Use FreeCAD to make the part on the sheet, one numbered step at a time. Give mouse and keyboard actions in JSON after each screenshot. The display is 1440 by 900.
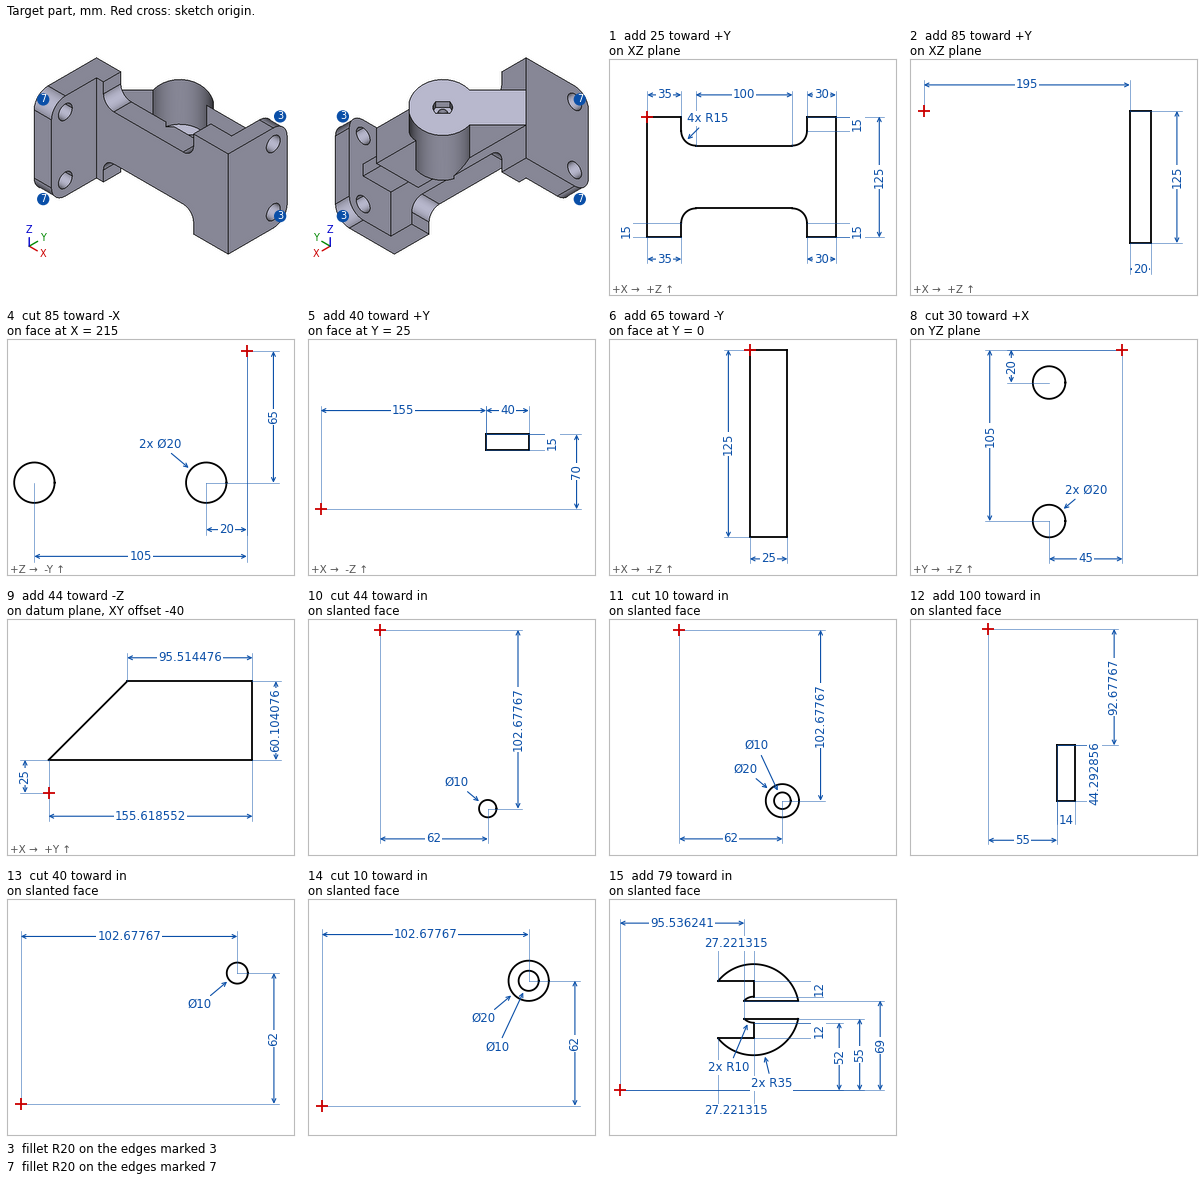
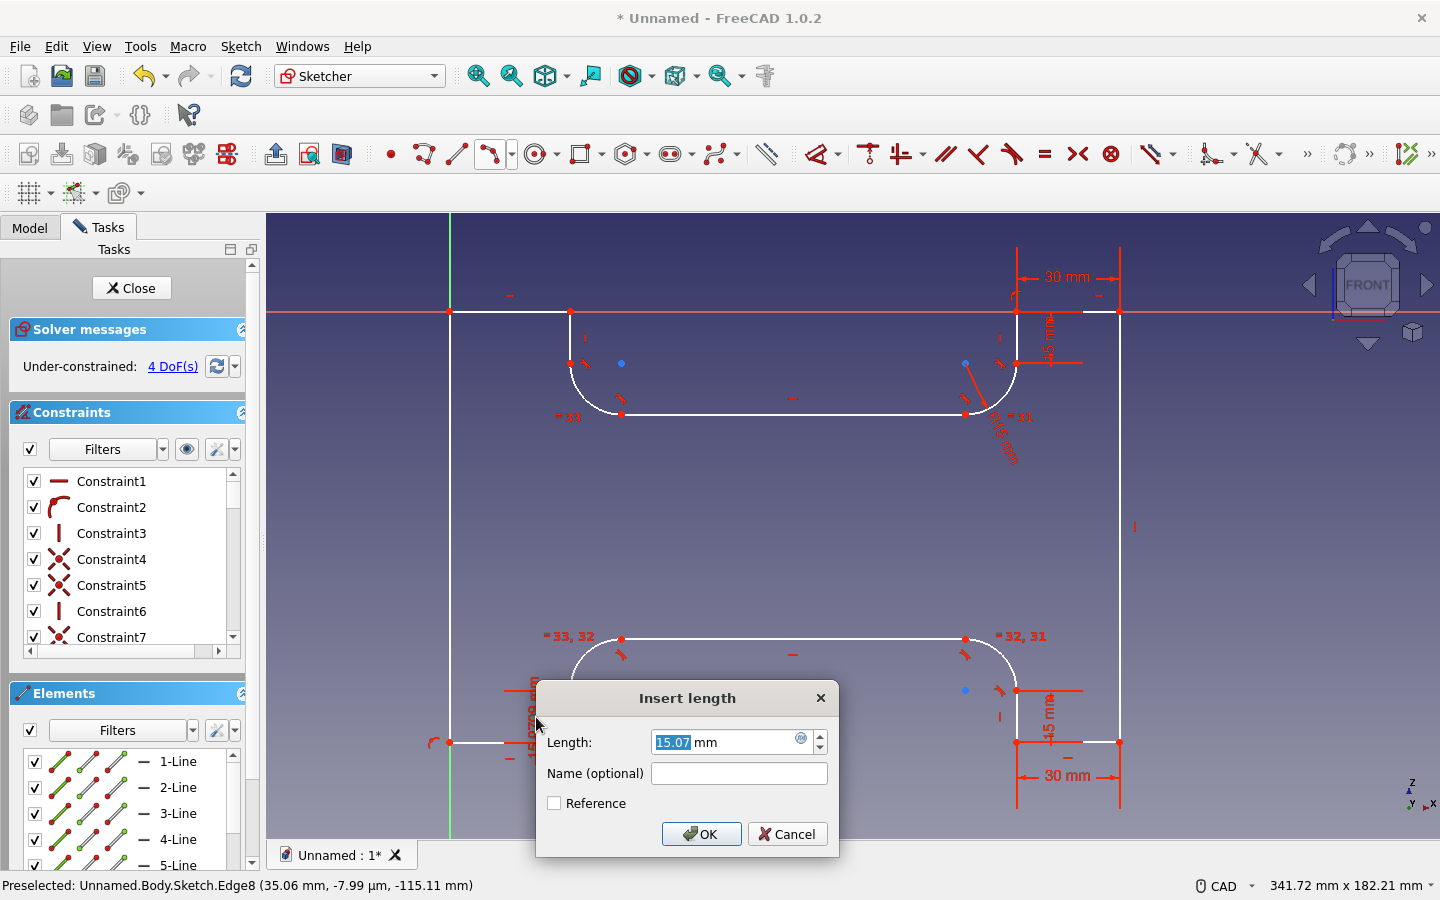
{"action": "type", "text": "15"}
{"action": "key", "text": "Return"}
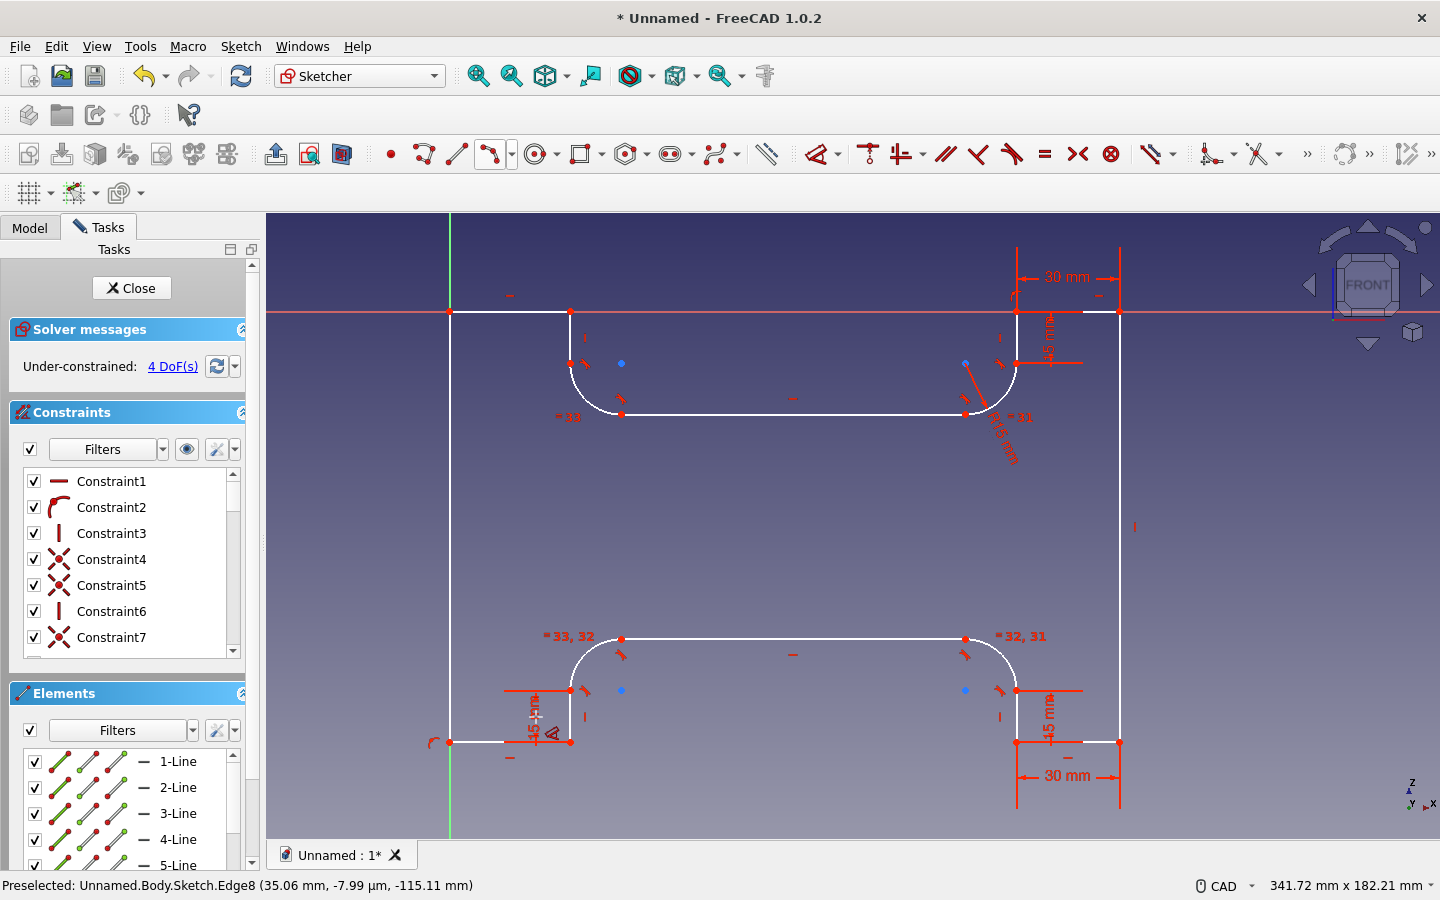
{"action": "left_click", "coordinate": [534, 742]}
{"action": "left_click", "coordinate": [510, 776]}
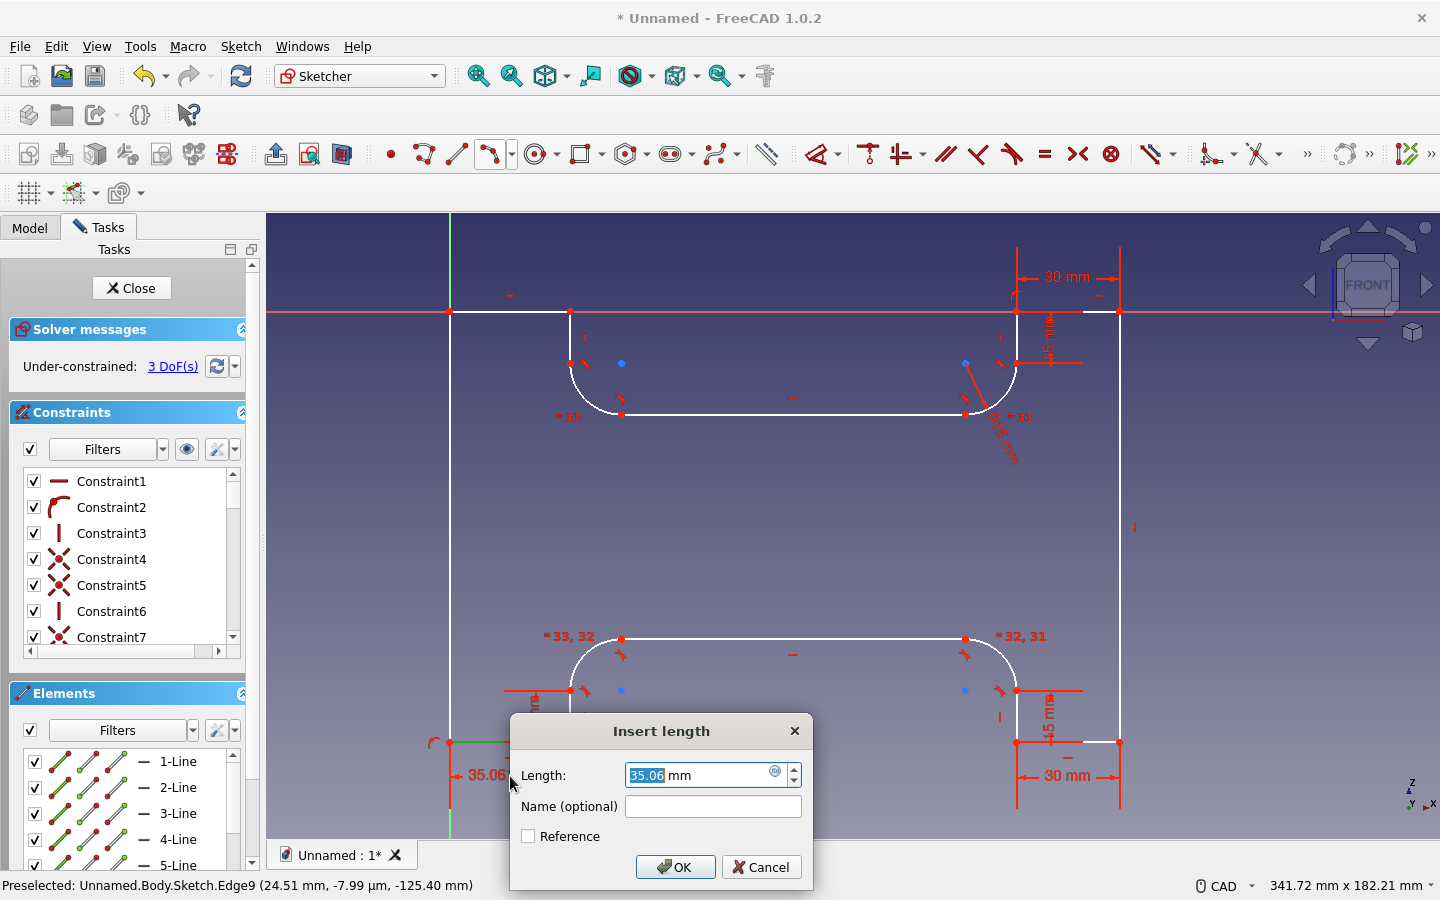
{"action": "type", "text": "35"}
{"action": "key", "text": "Return"}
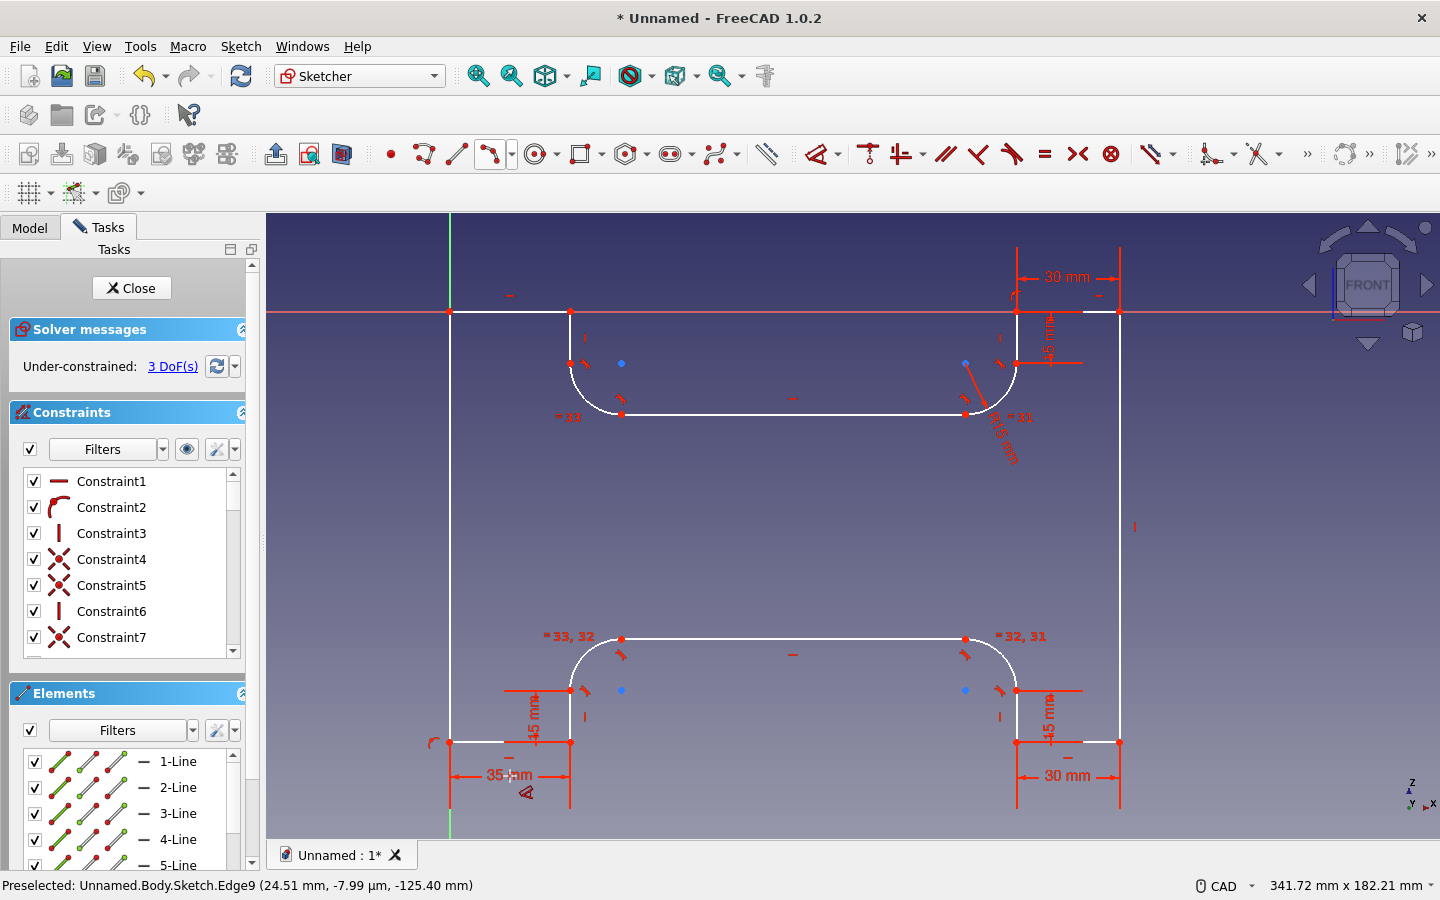
{"action": "left_click", "coordinate": [486, 312]}
{"action": "left_click", "coordinate": [510, 278]}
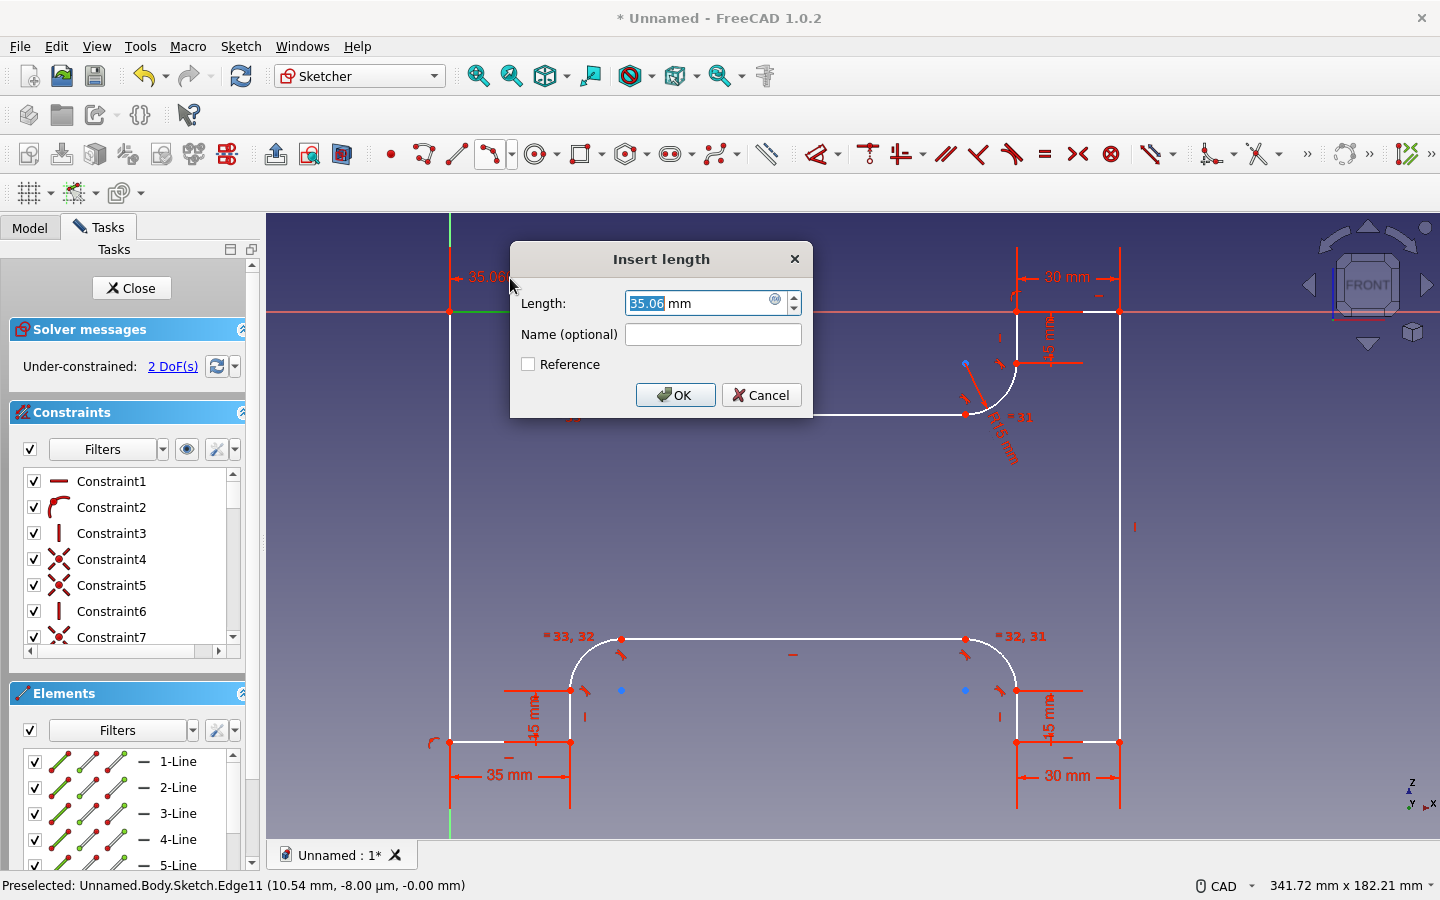
{"action": "type", "text": "35"}
{"action": "key", "text": "Return"}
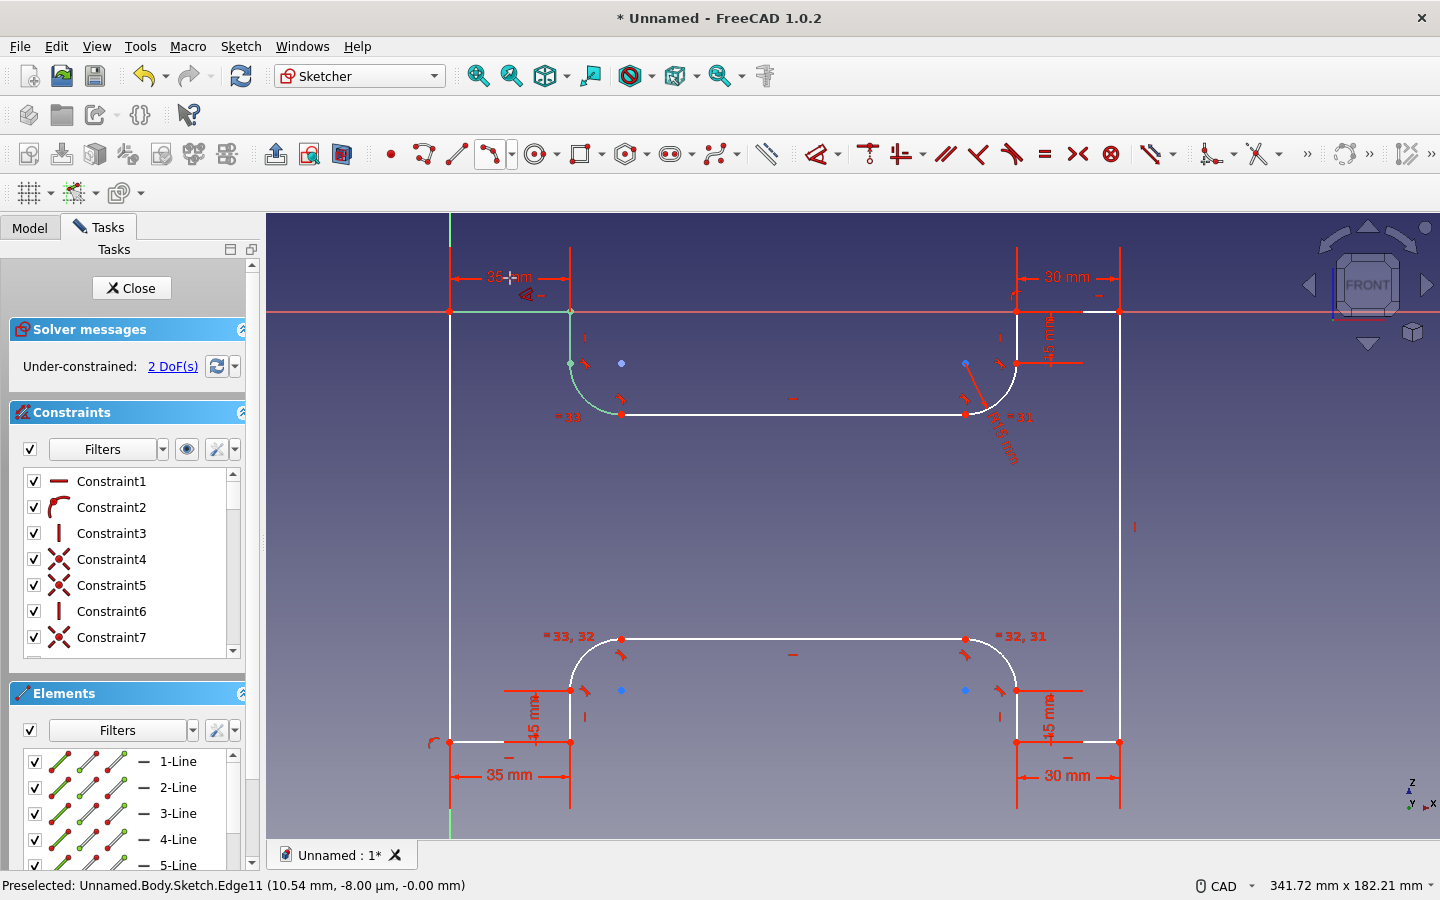
{"action": "left_click", "coordinate": [725, 415]}
{"action": "left_click", "coordinate": [793, 381]}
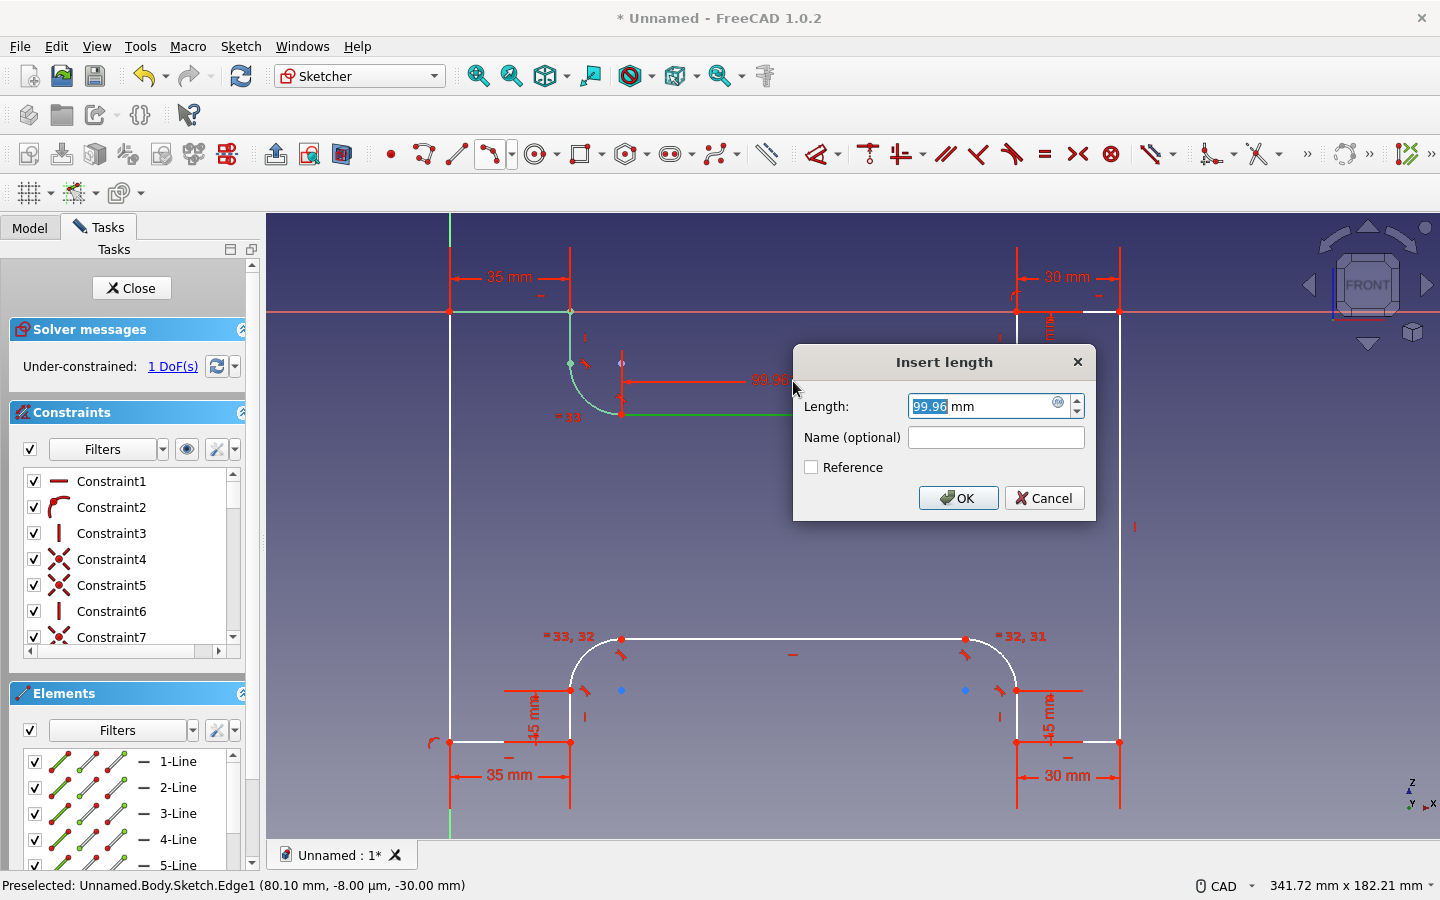
{"action": "type", "text": "100"}
{"action": "key", "text": "Return"}